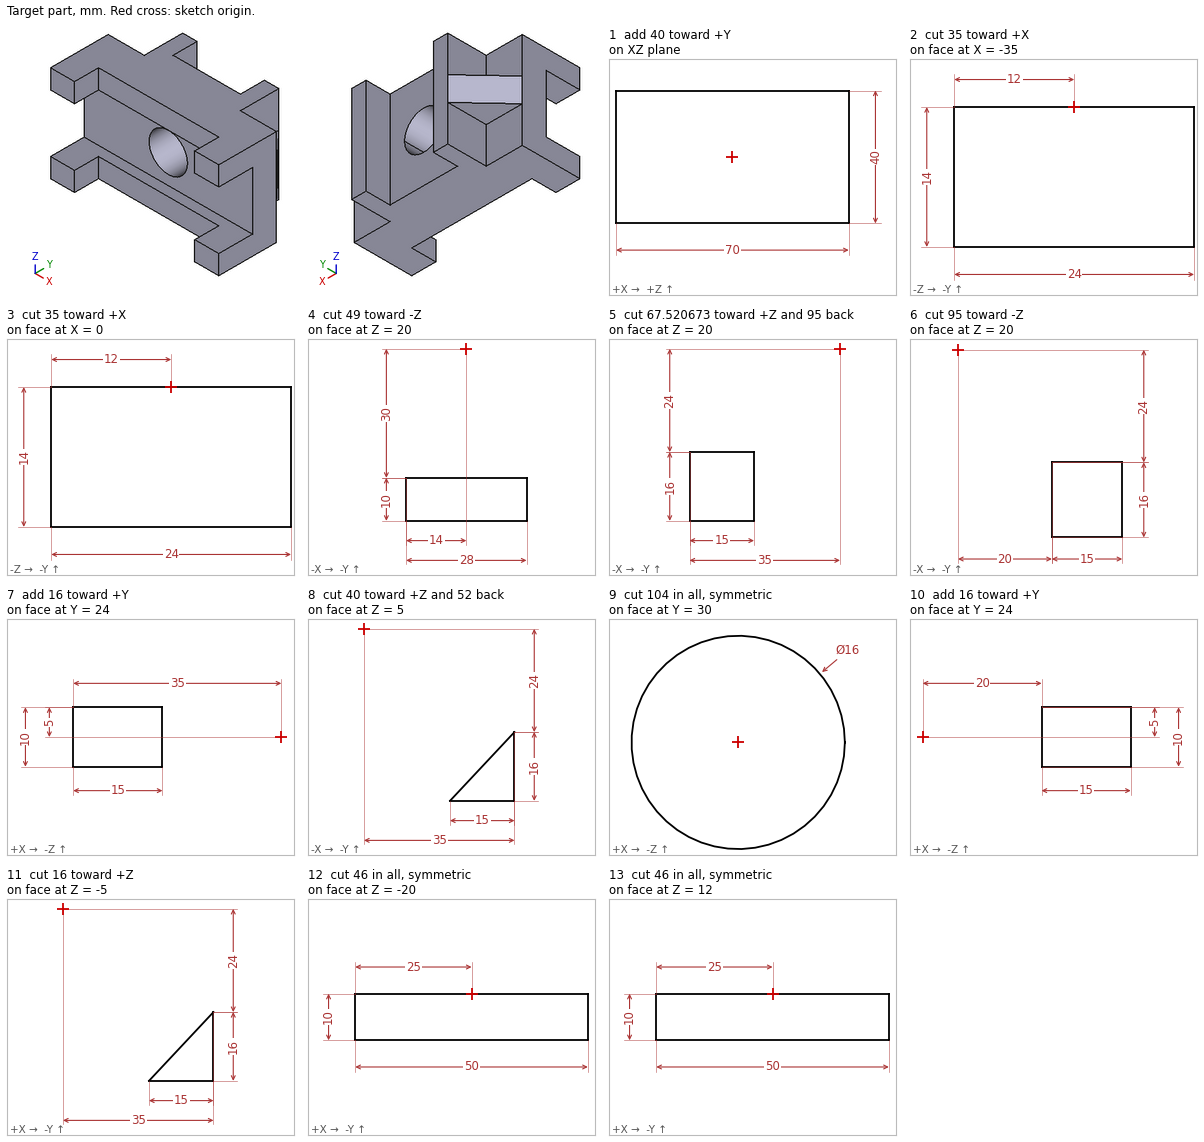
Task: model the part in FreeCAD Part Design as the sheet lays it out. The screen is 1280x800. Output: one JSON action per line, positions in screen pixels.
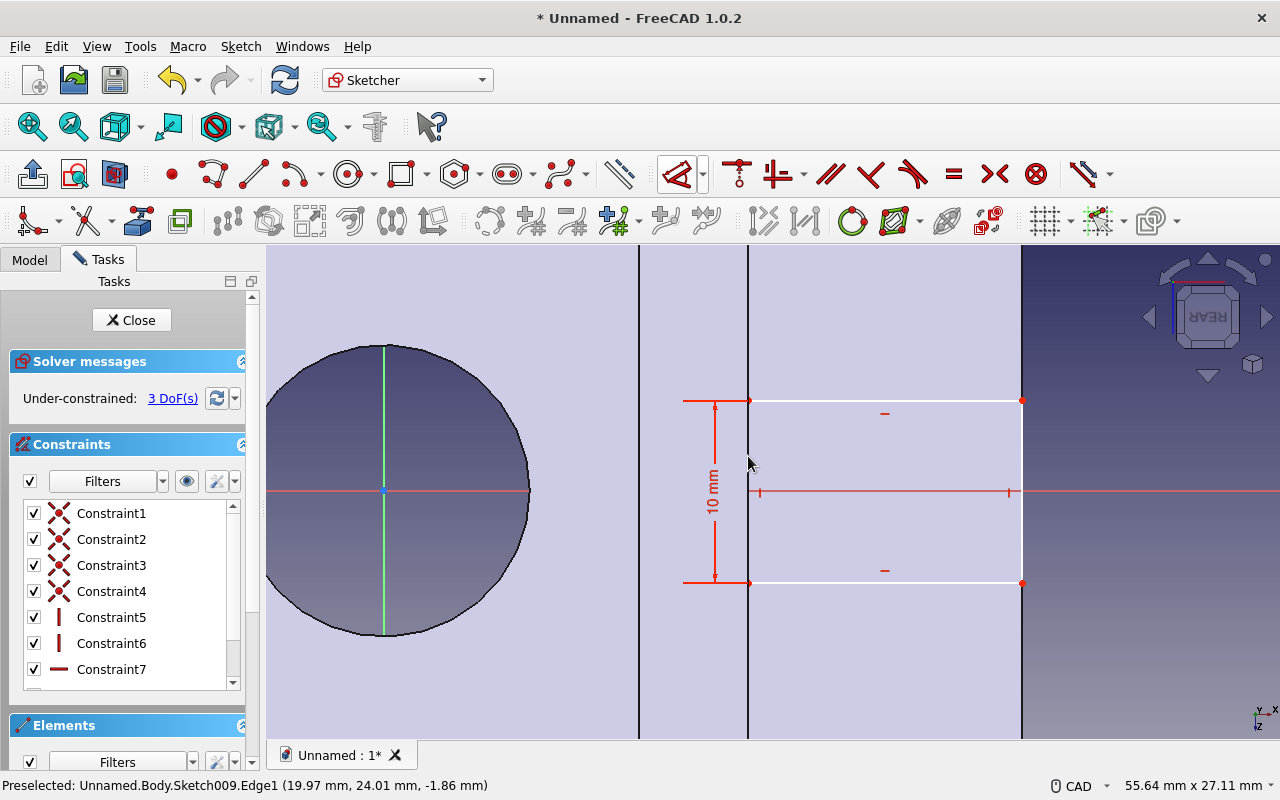
{"action": "left_click", "coordinate": [830, 583]}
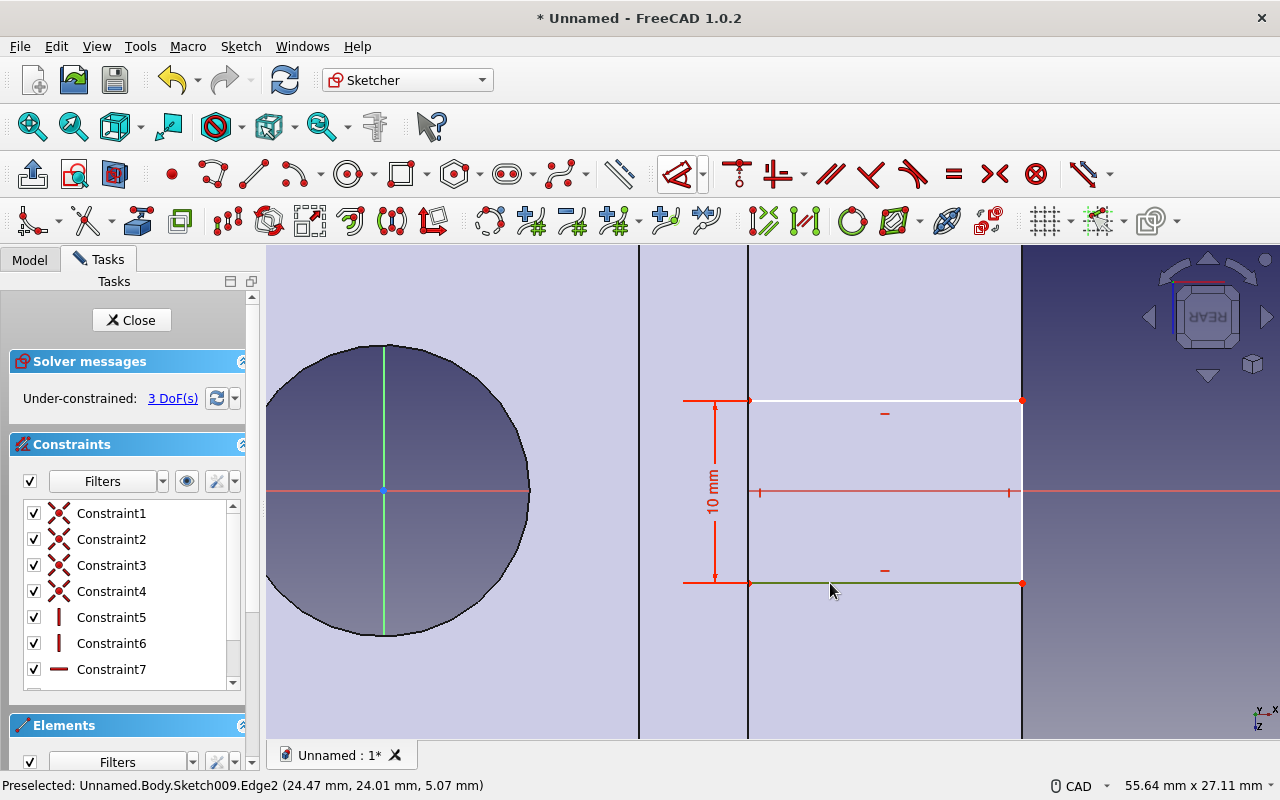
{"action": "key", "text": "l"}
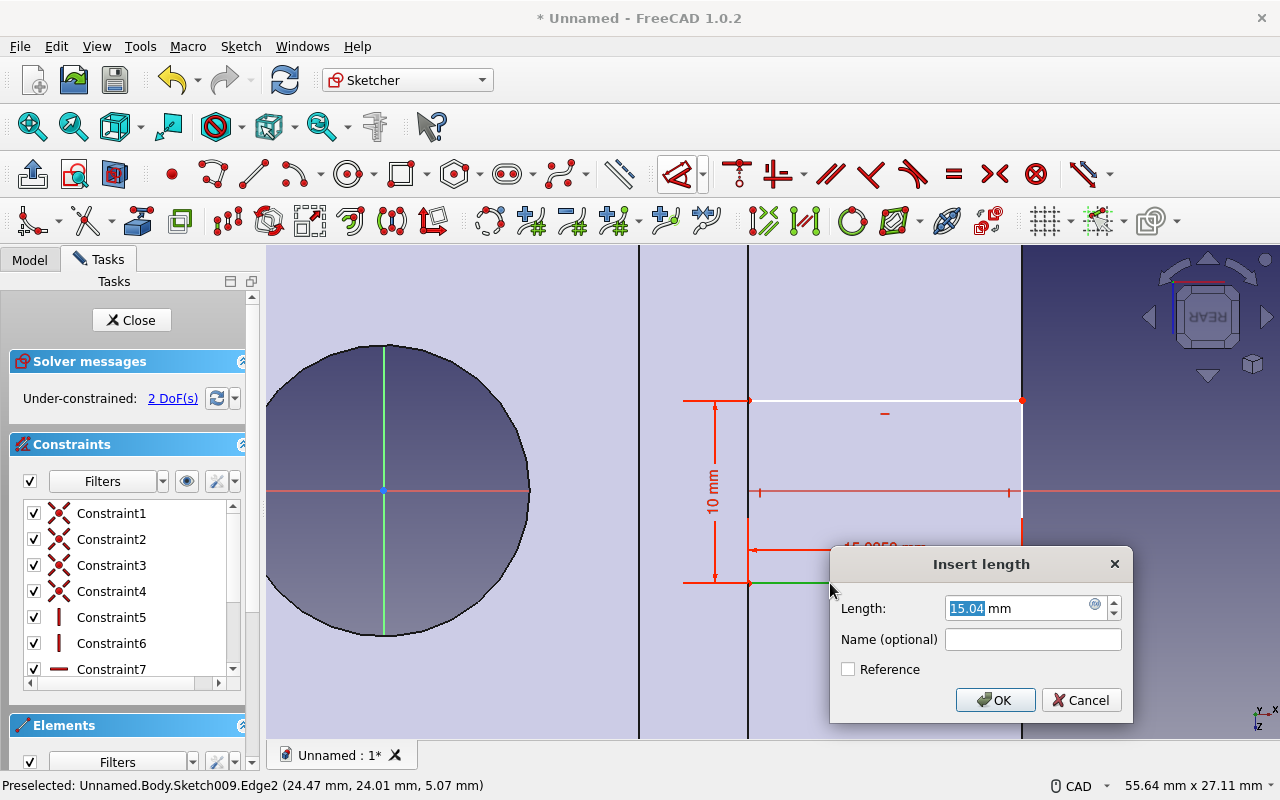
{"action": "type", "text": "15"}
{"action": "key", "text": "Return"}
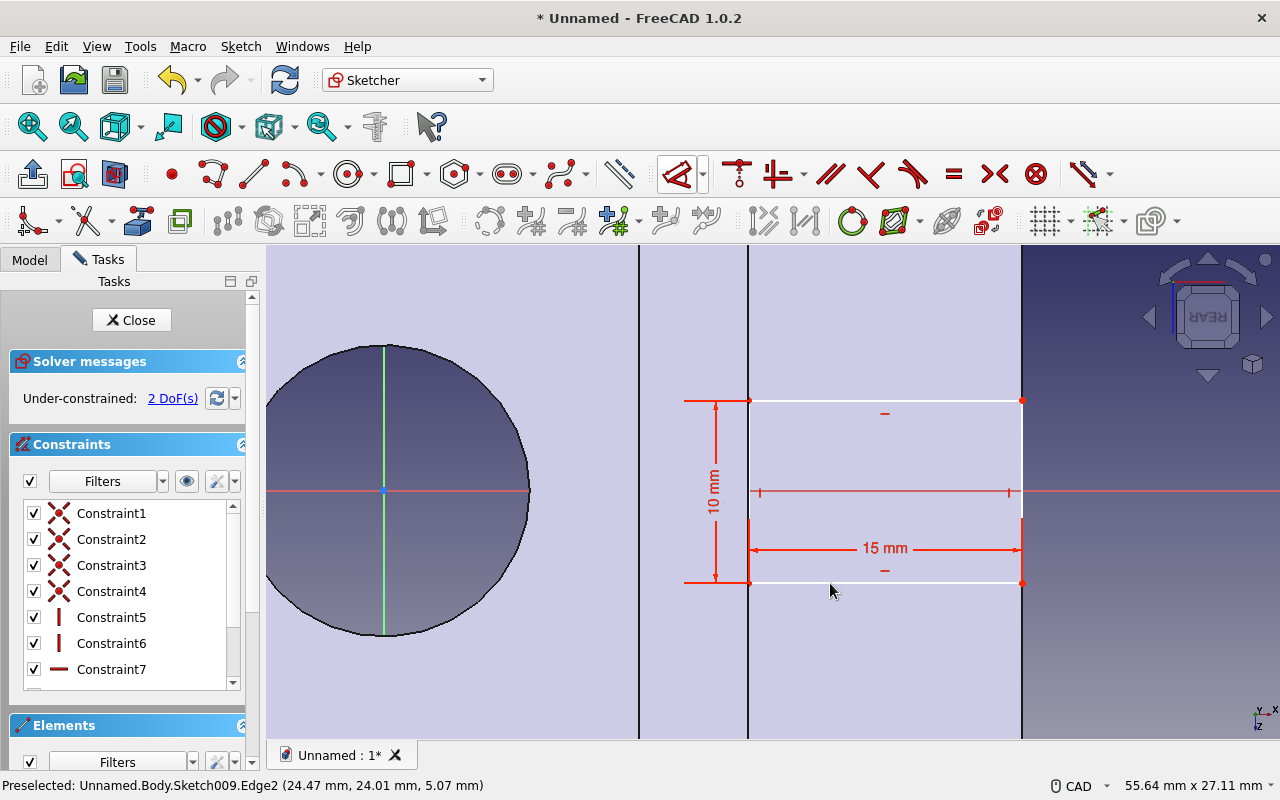
{"action": "left_click", "coordinate": [749, 401]}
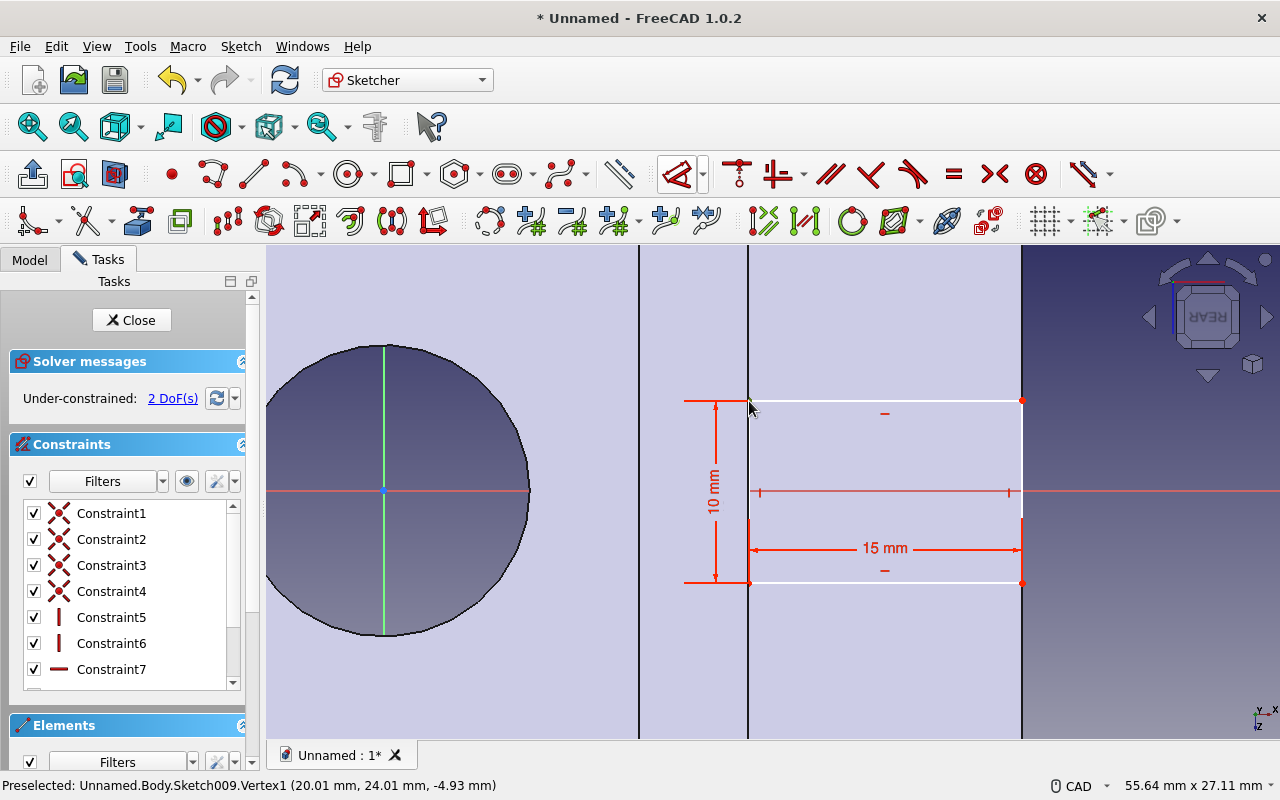
{"action": "key", "text": "i"}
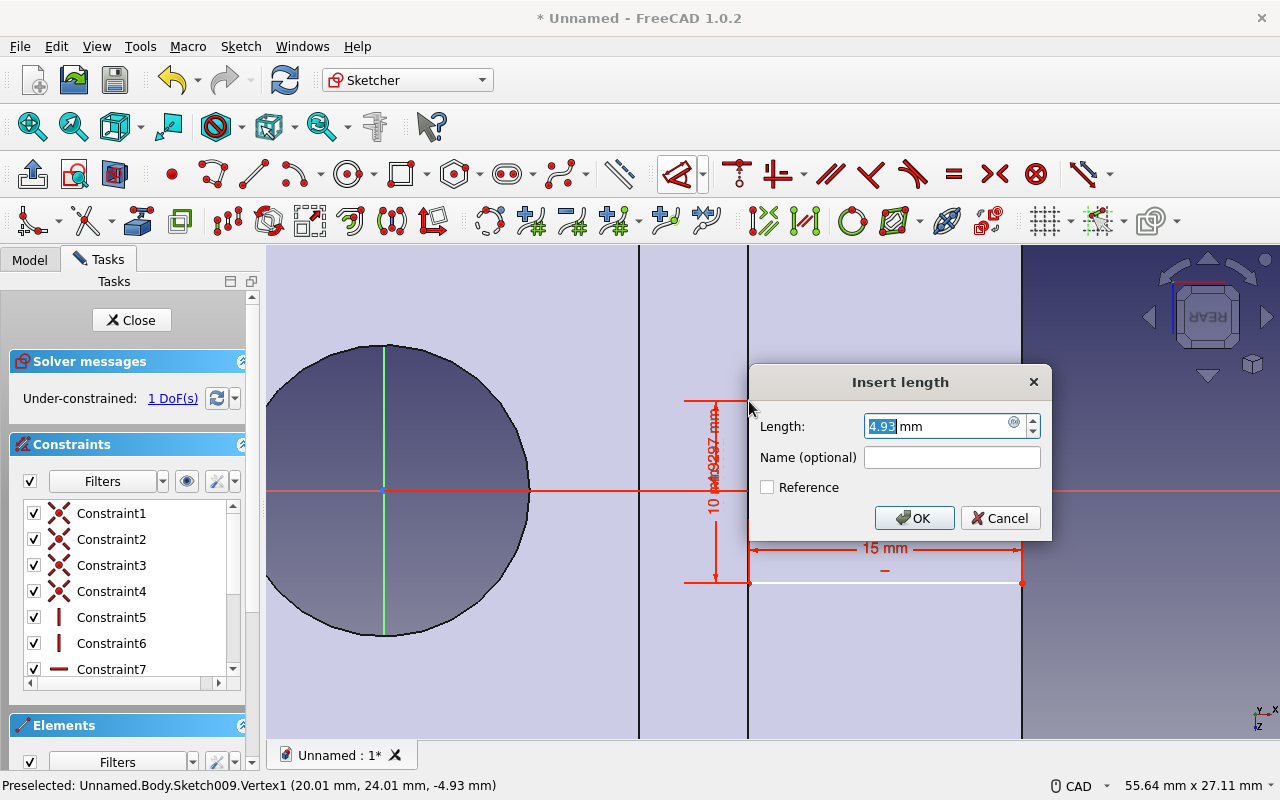
{"action": "type", "text": "5"}
{"action": "key", "text": "Return"}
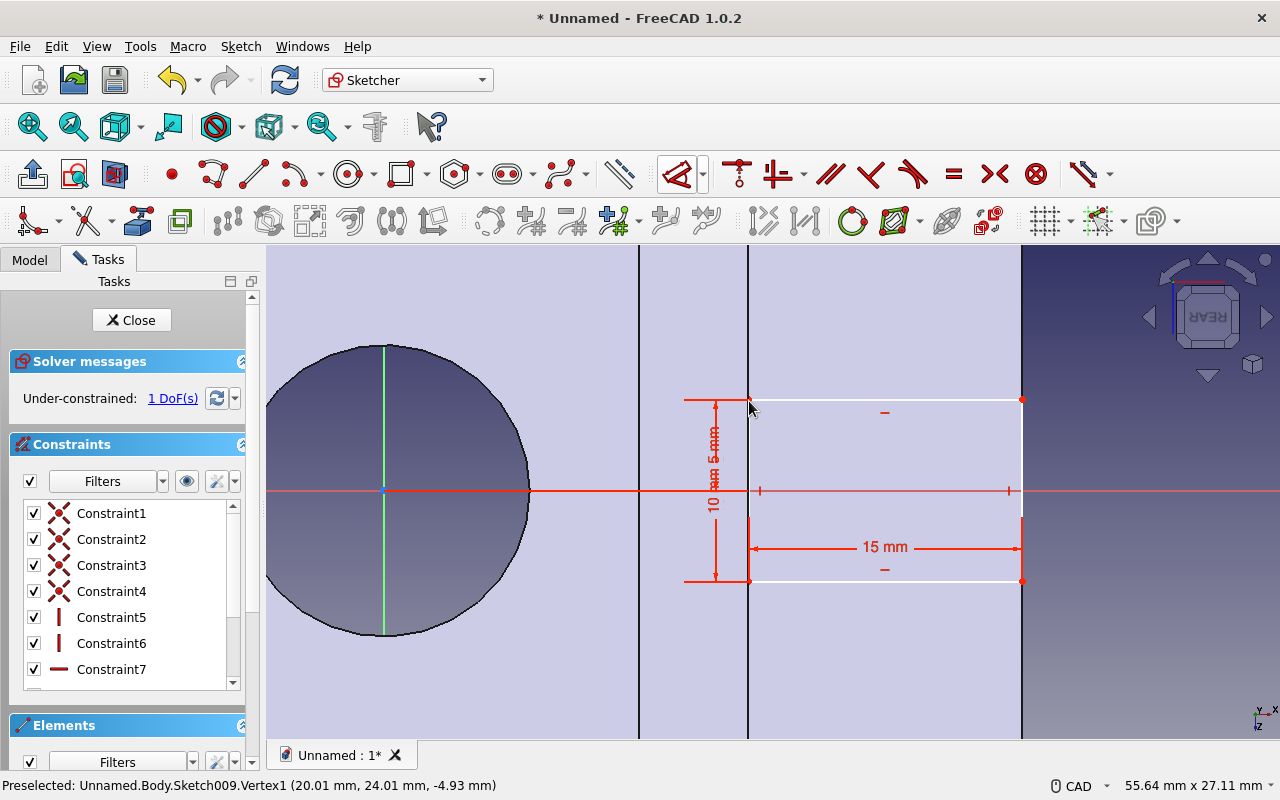
{"action": "left_click", "coordinate": [749, 400]}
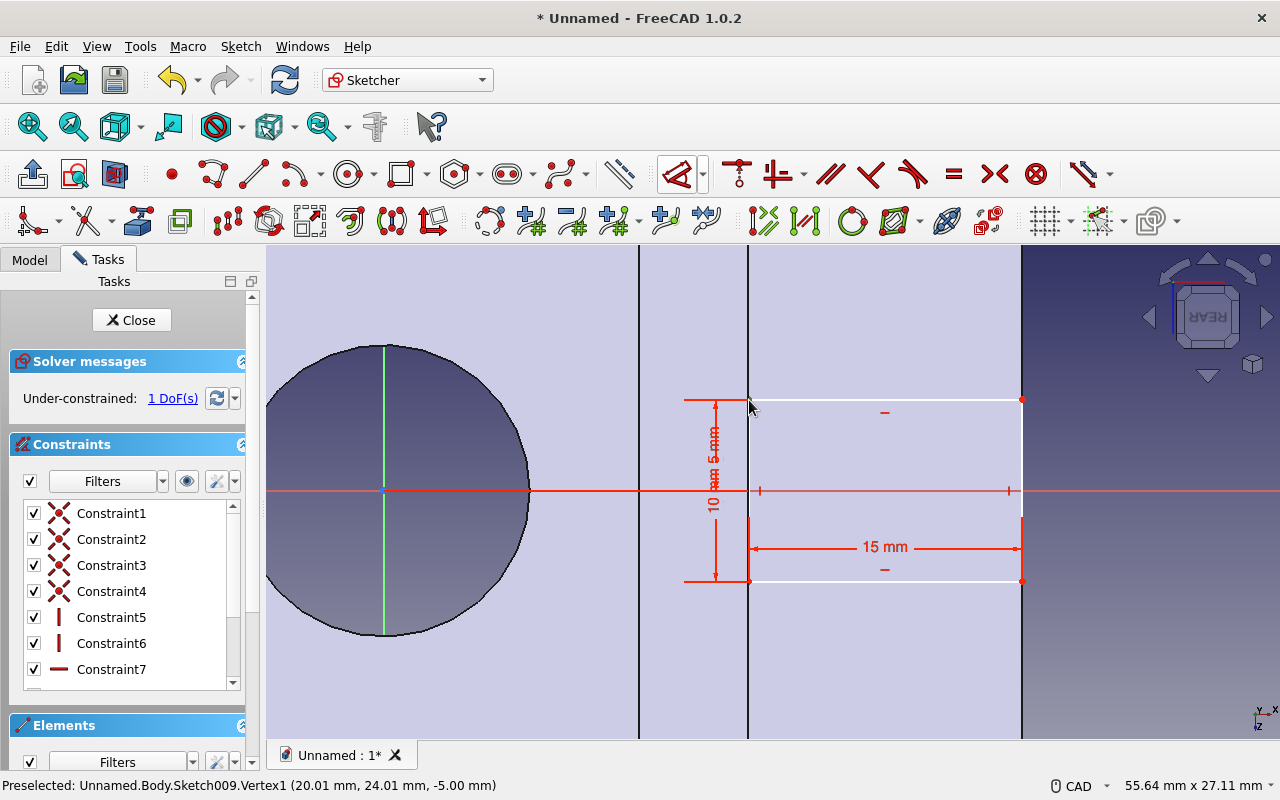
{"action": "key", "text": "l"}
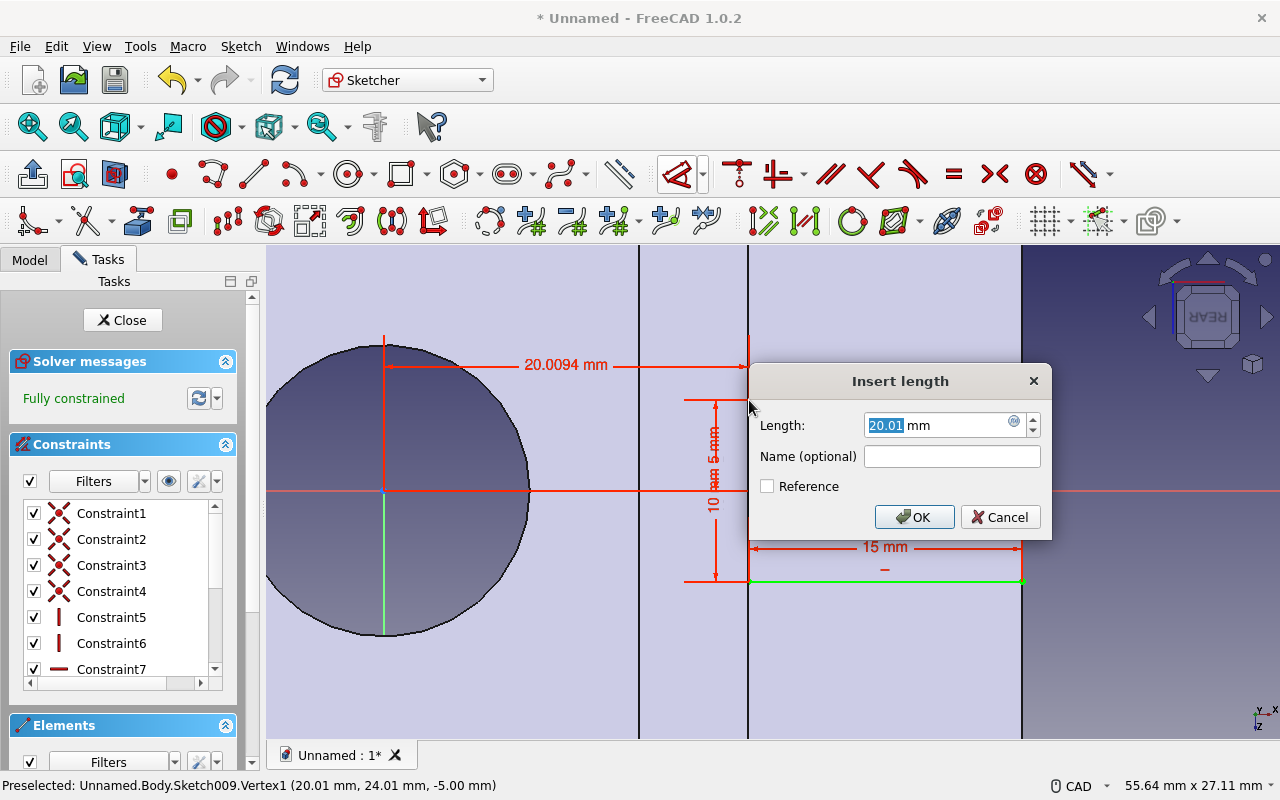
{"action": "type", "text": "20"}
{"action": "key", "text": "Return"}